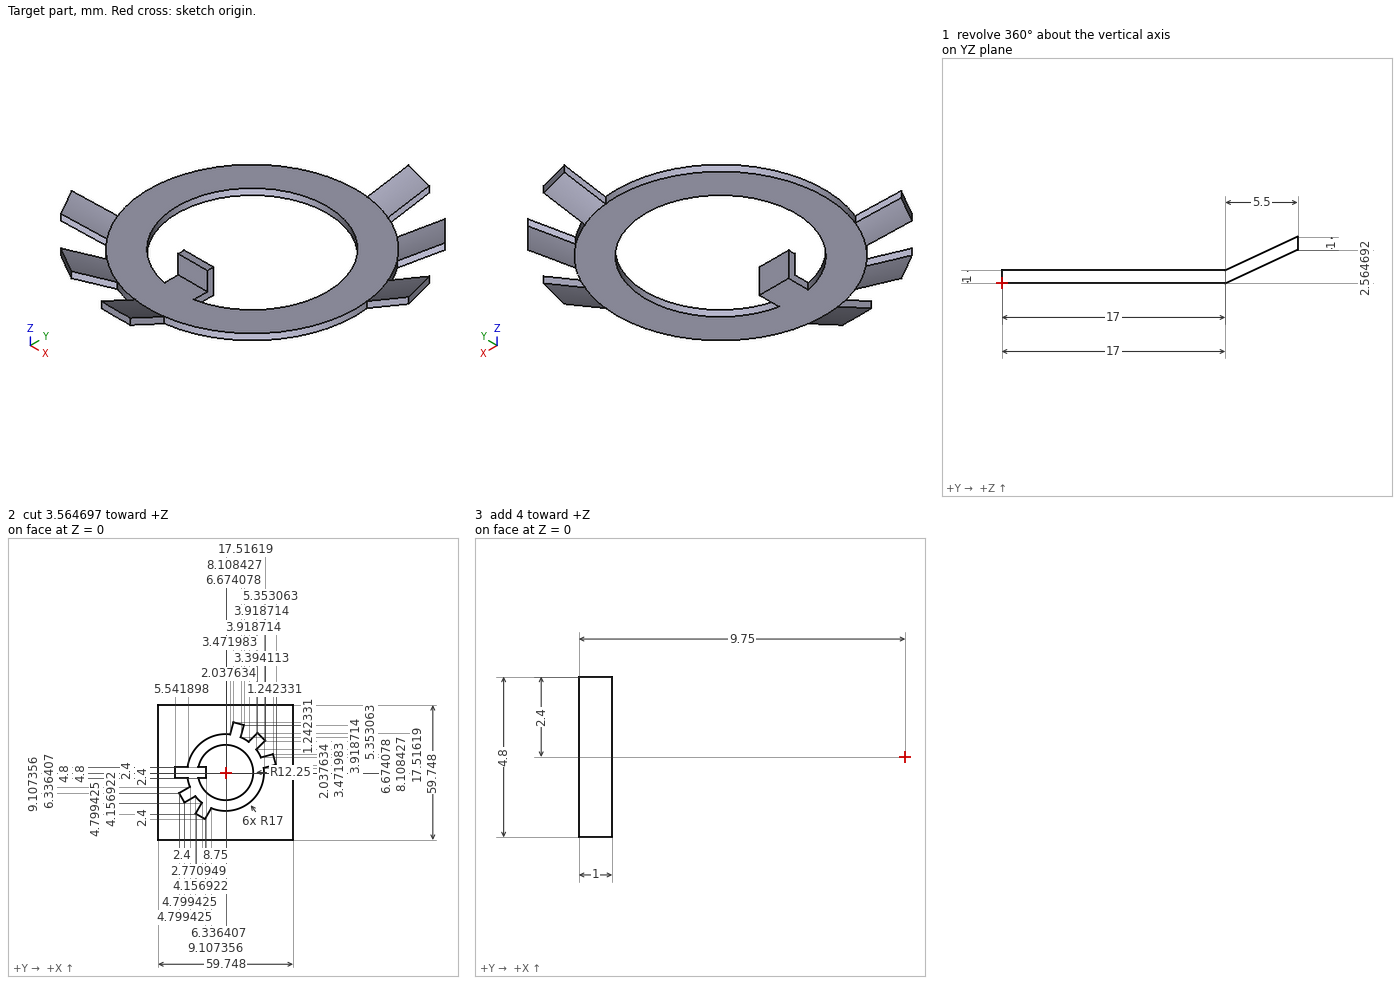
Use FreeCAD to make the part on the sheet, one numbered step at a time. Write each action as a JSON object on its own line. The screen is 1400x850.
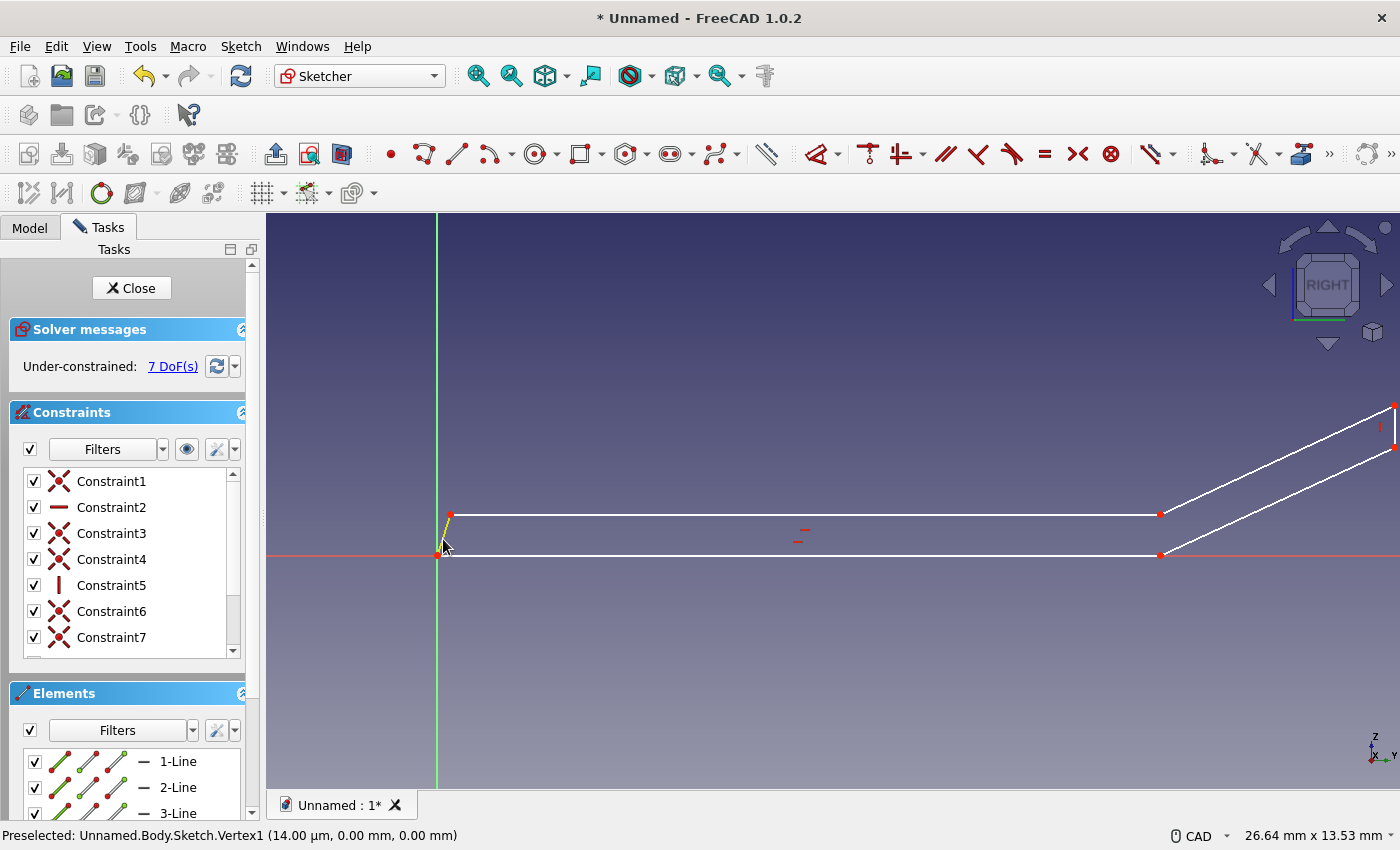
{"action": "left_click", "coordinate": [443, 539]}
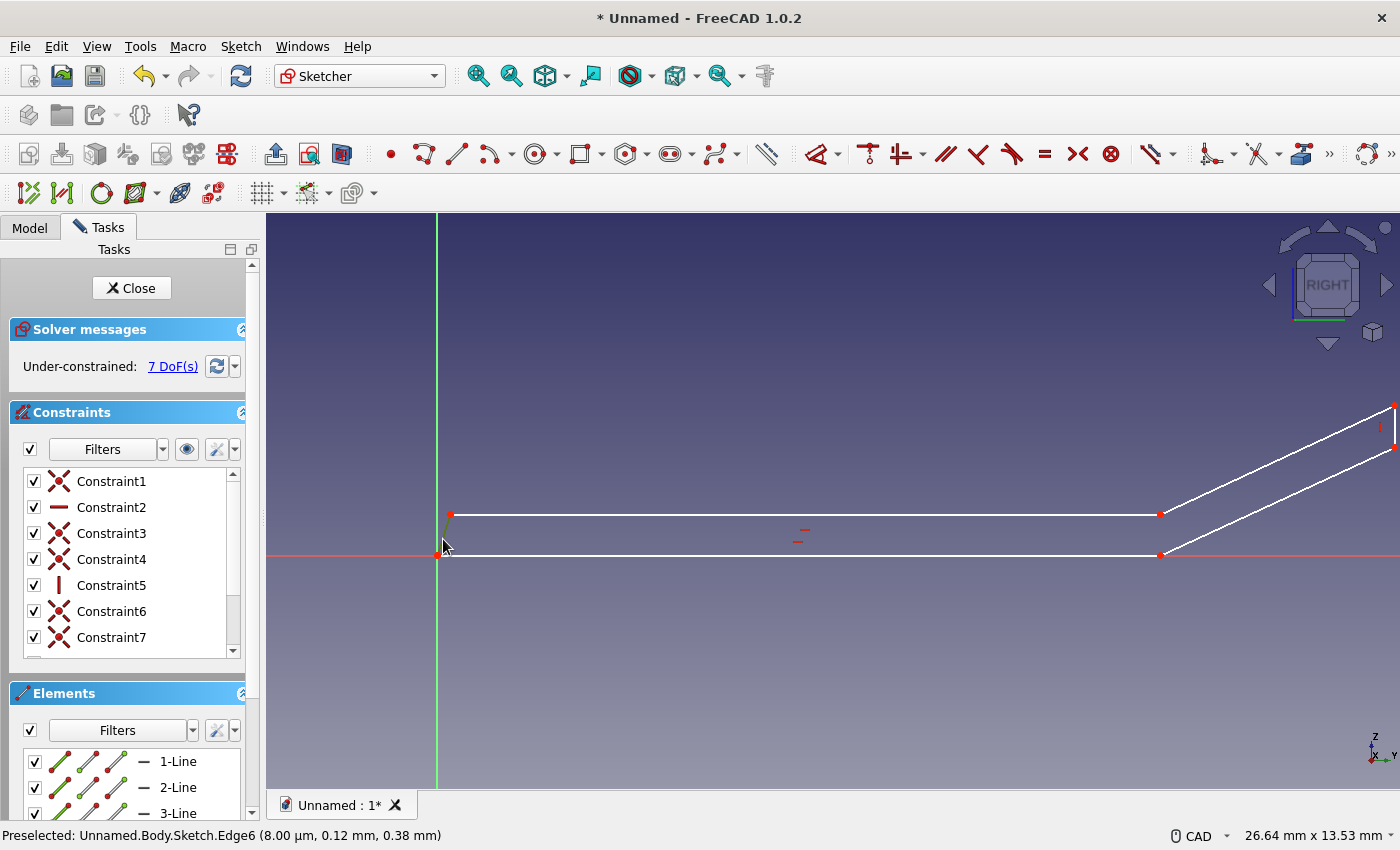
{"action": "left_click", "coordinate": [922, 154]}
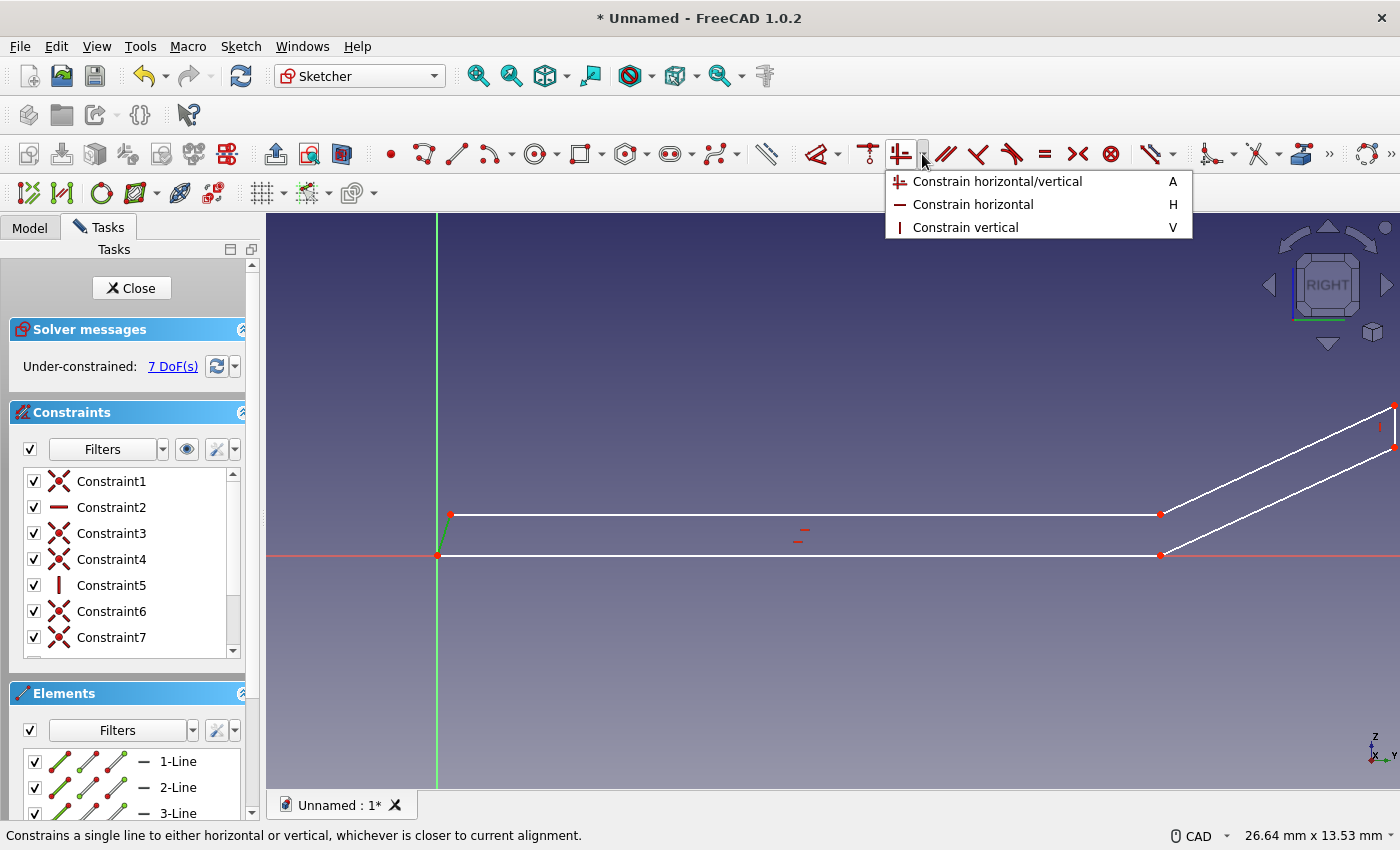
{"action": "left_click", "coordinate": [1039, 228]}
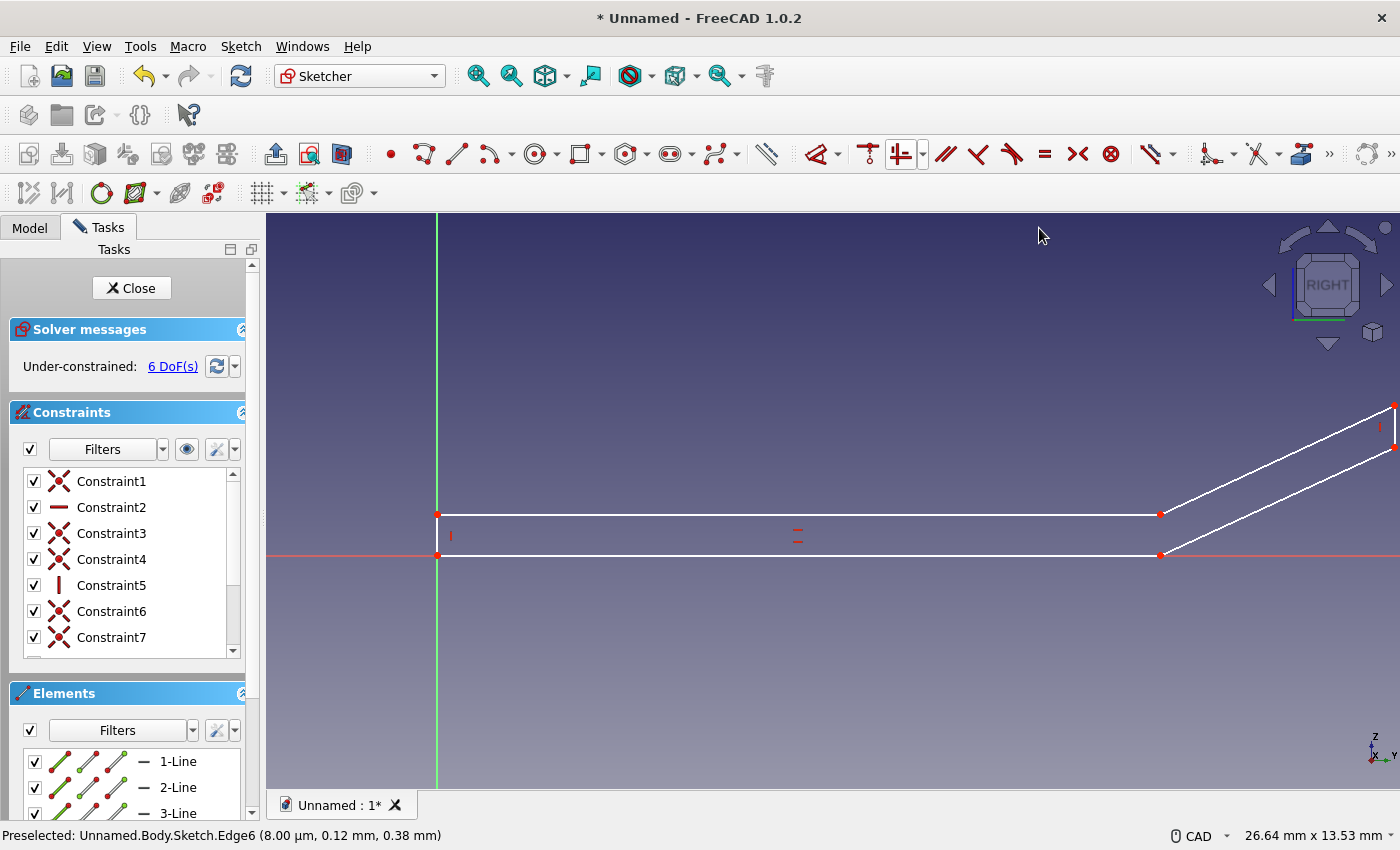
{"action": "scroll", "coordinate": [456, 544], "scroll_direction": "down", "scroll_amount": 2}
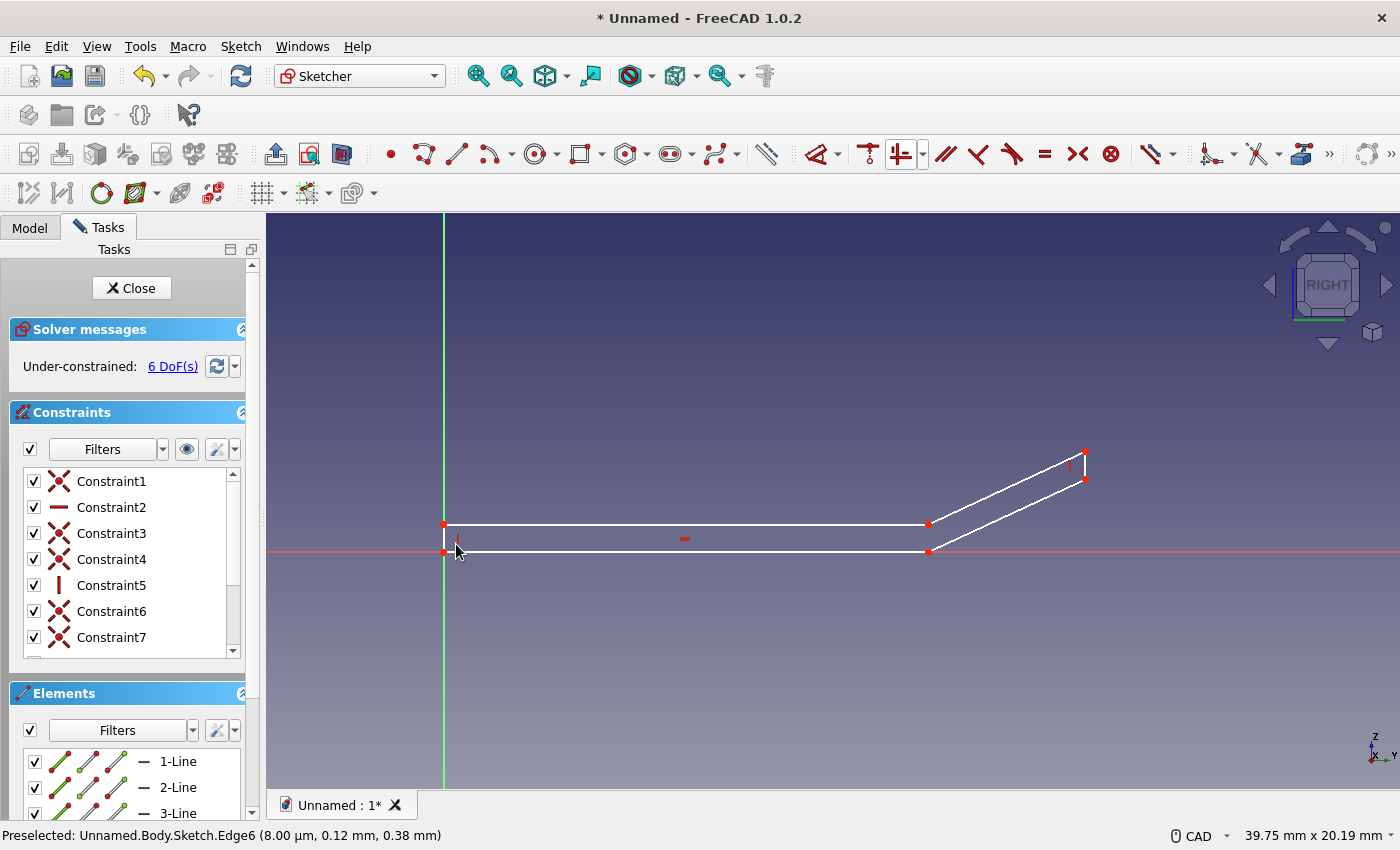
{"action": "scroll", "coordinate": [1085, 471], "scroll_direction": "up", "scroll_amount": 3}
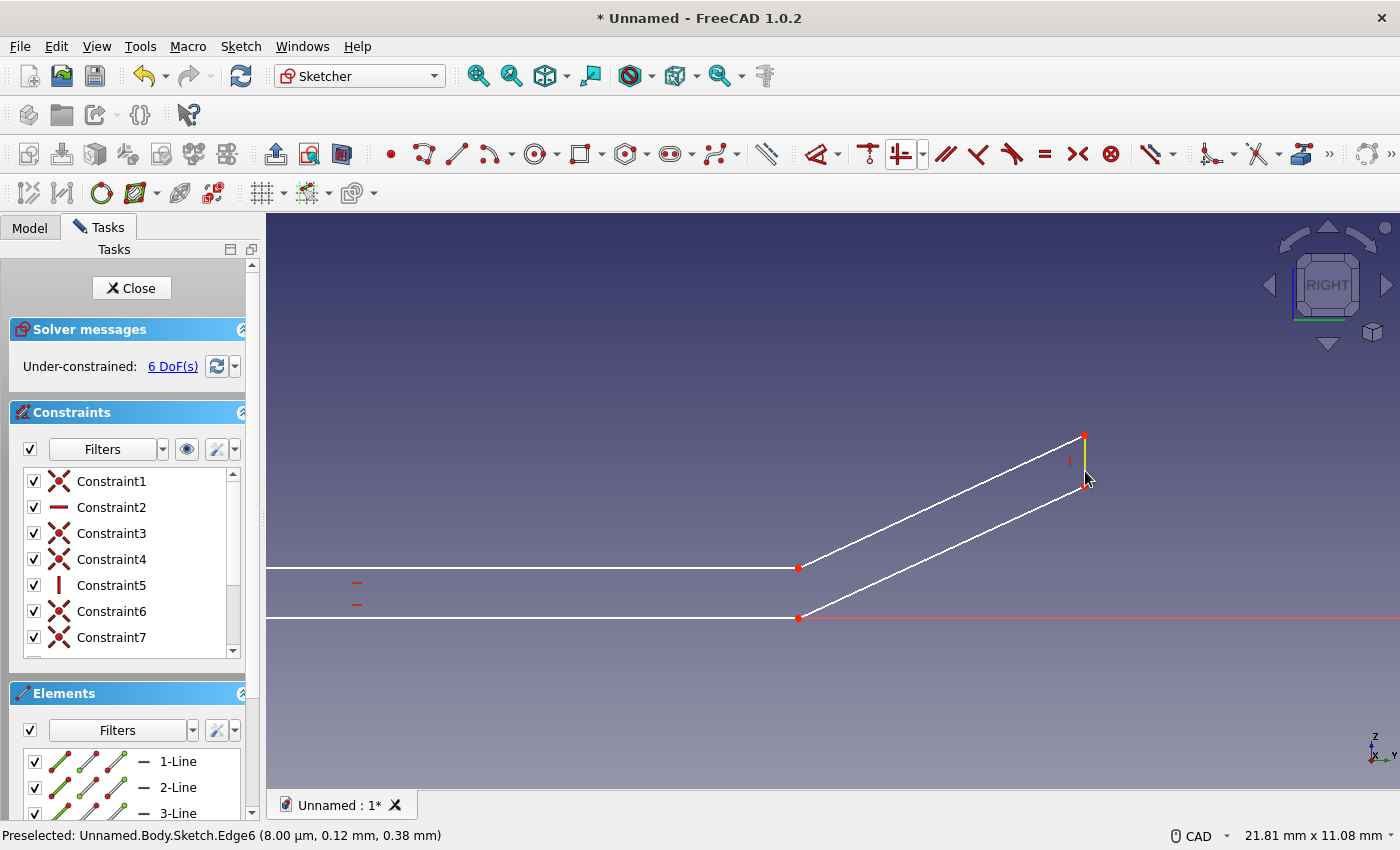
{"action": "left_click", "coordinate": [1085, 471]}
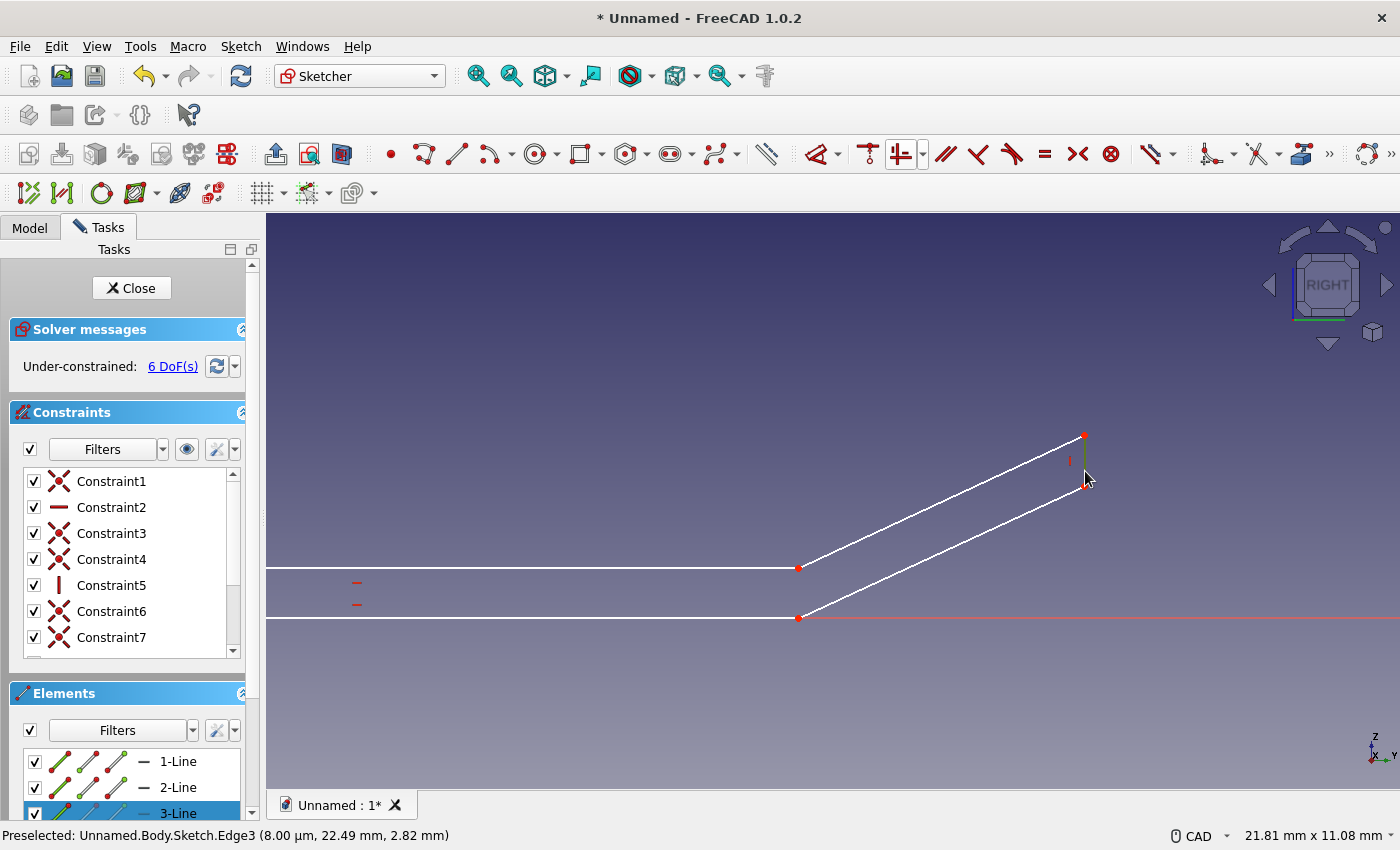
{"action": "key", "text": "i"}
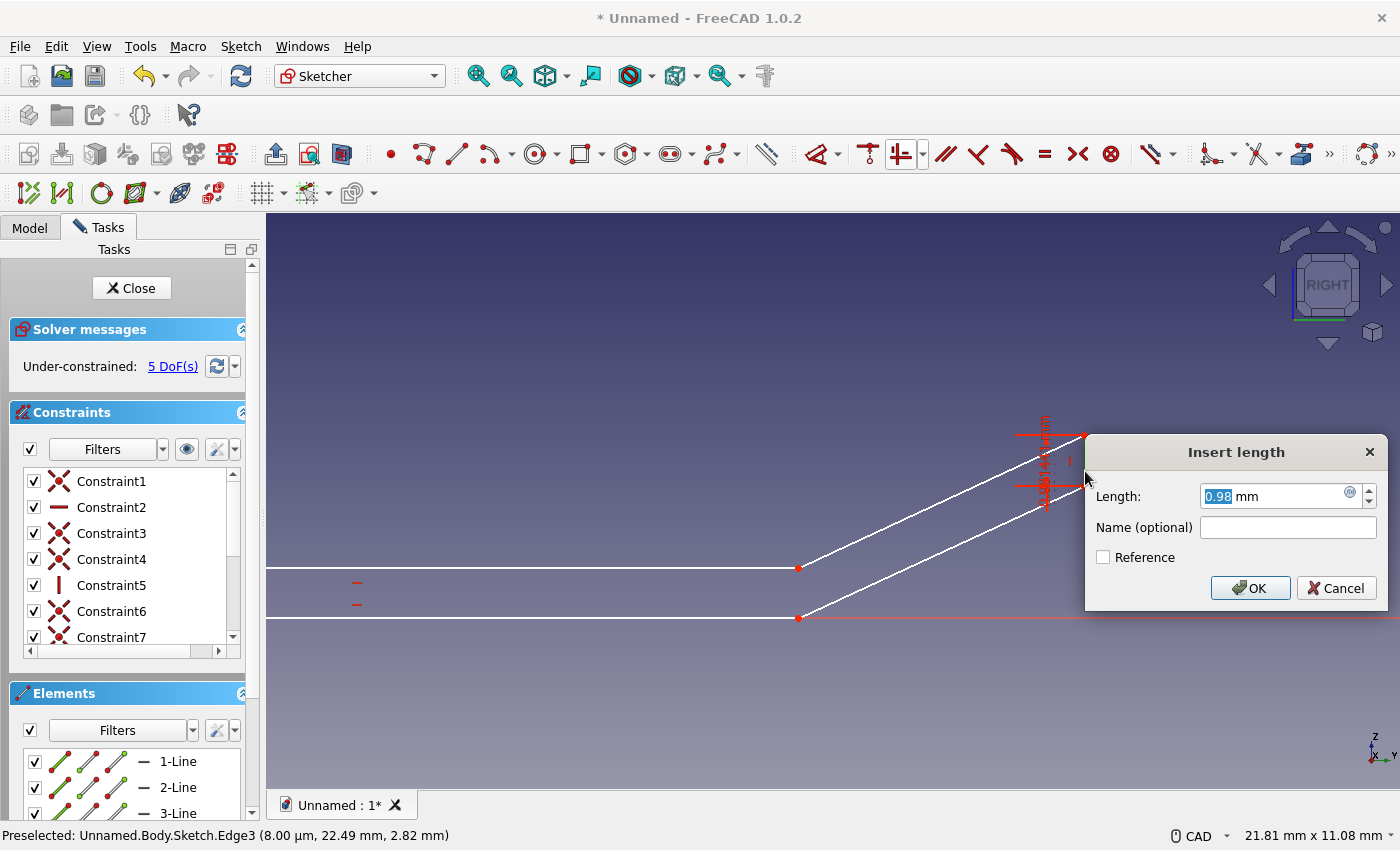
{"action": "type", "text": "1"}
{"action": "key", "text": "Return"}